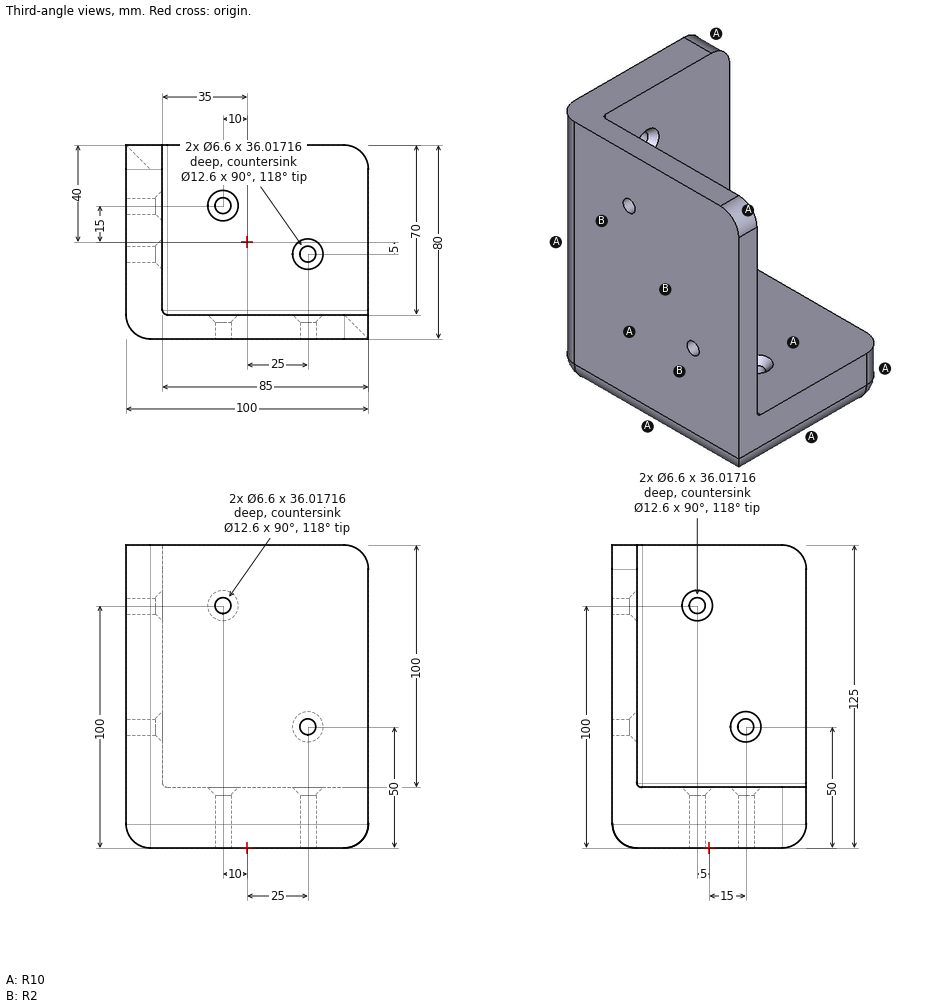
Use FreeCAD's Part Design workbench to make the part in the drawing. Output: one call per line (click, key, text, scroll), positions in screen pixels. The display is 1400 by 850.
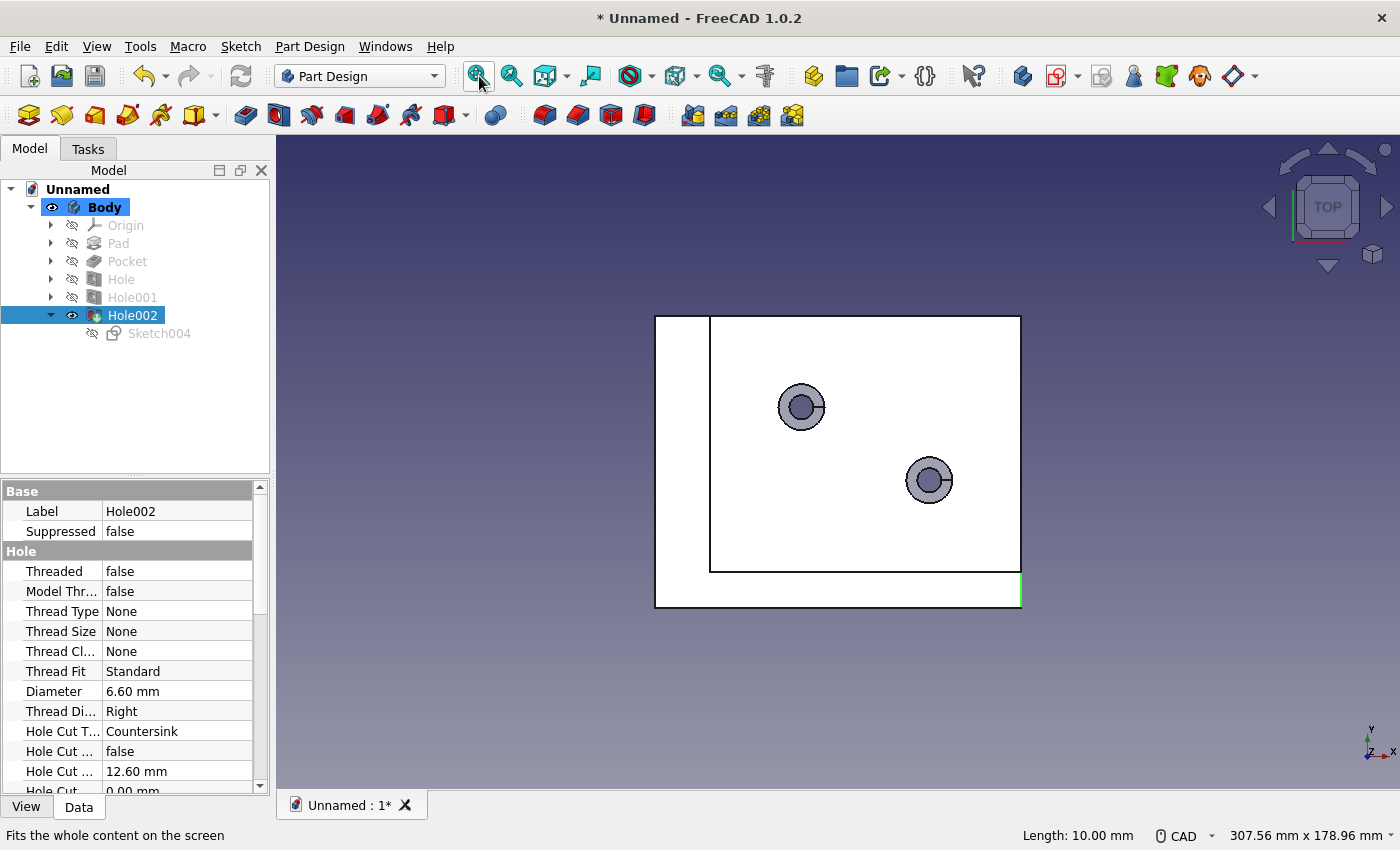
click(683, 315, ctrl)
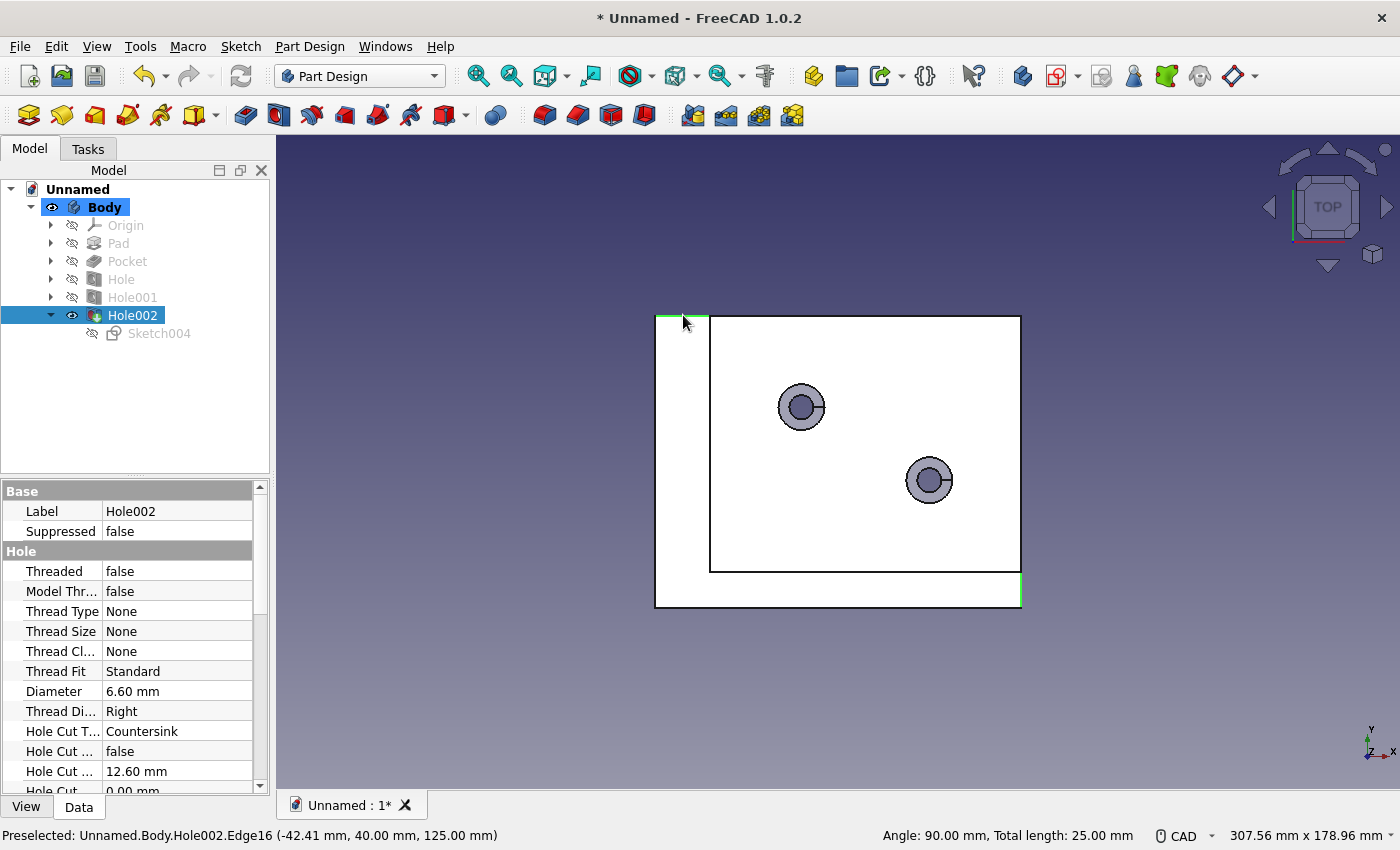
key(0)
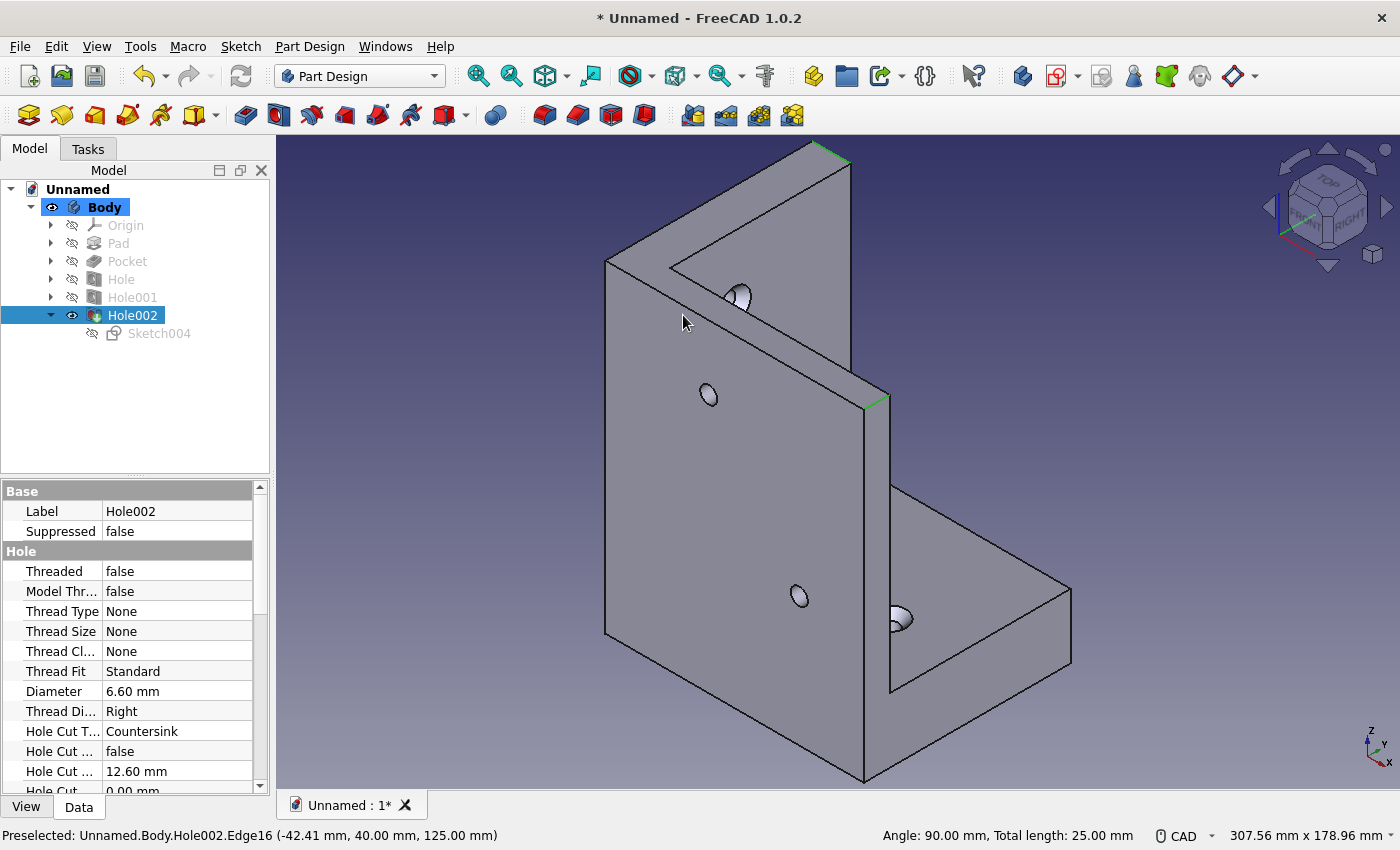
key(1)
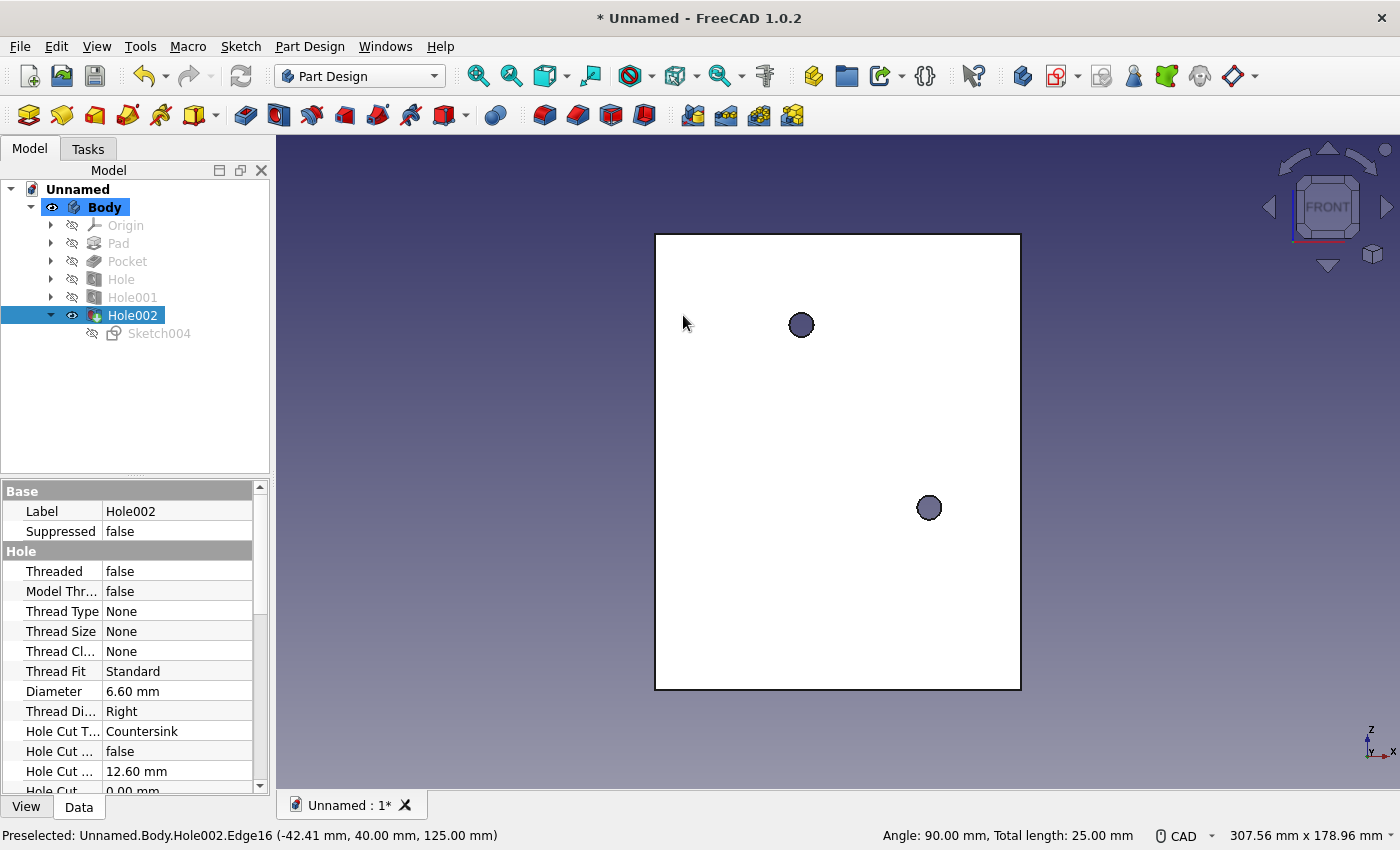
click(838, 689, ctrl)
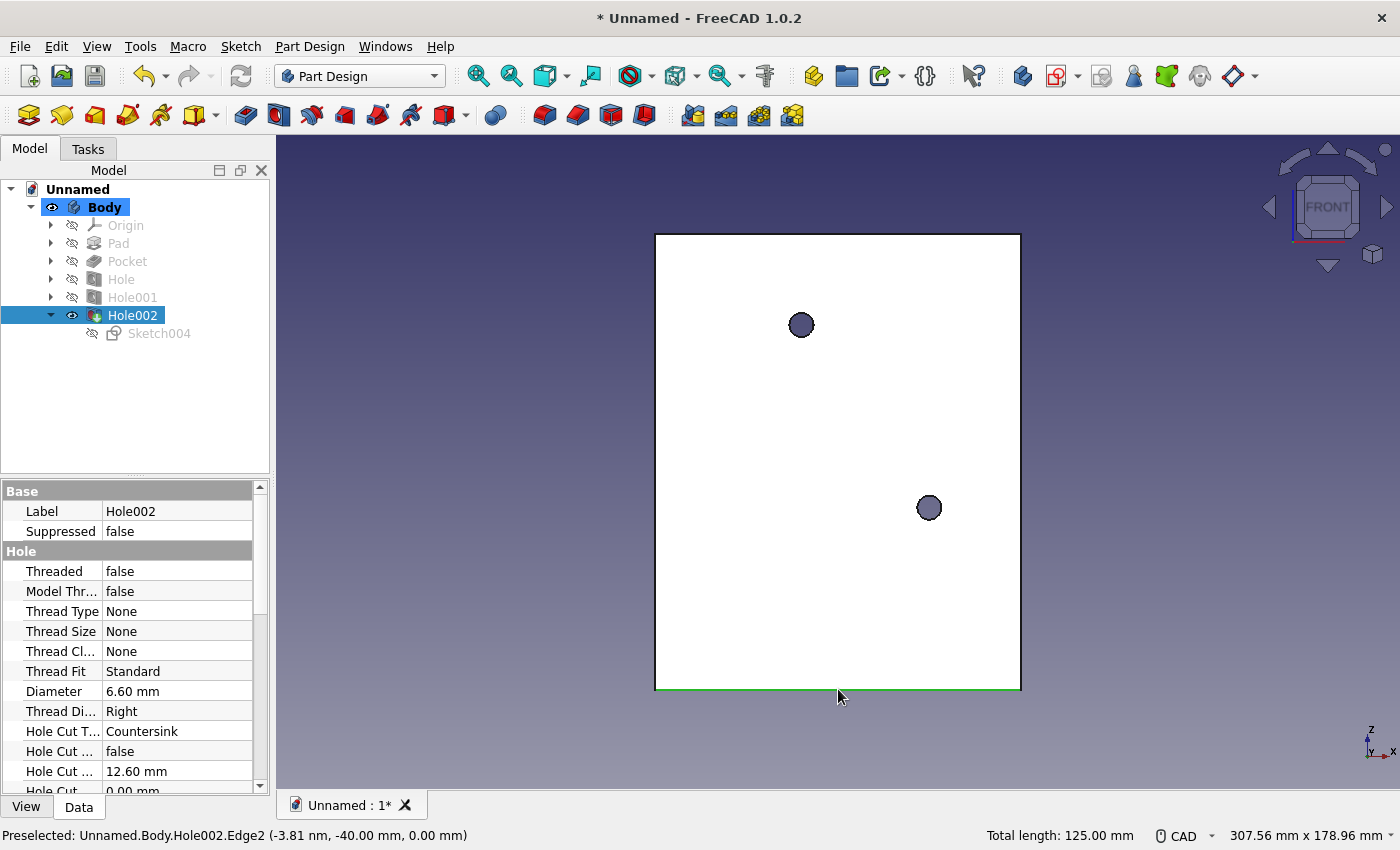
click(655, 461, ctrl)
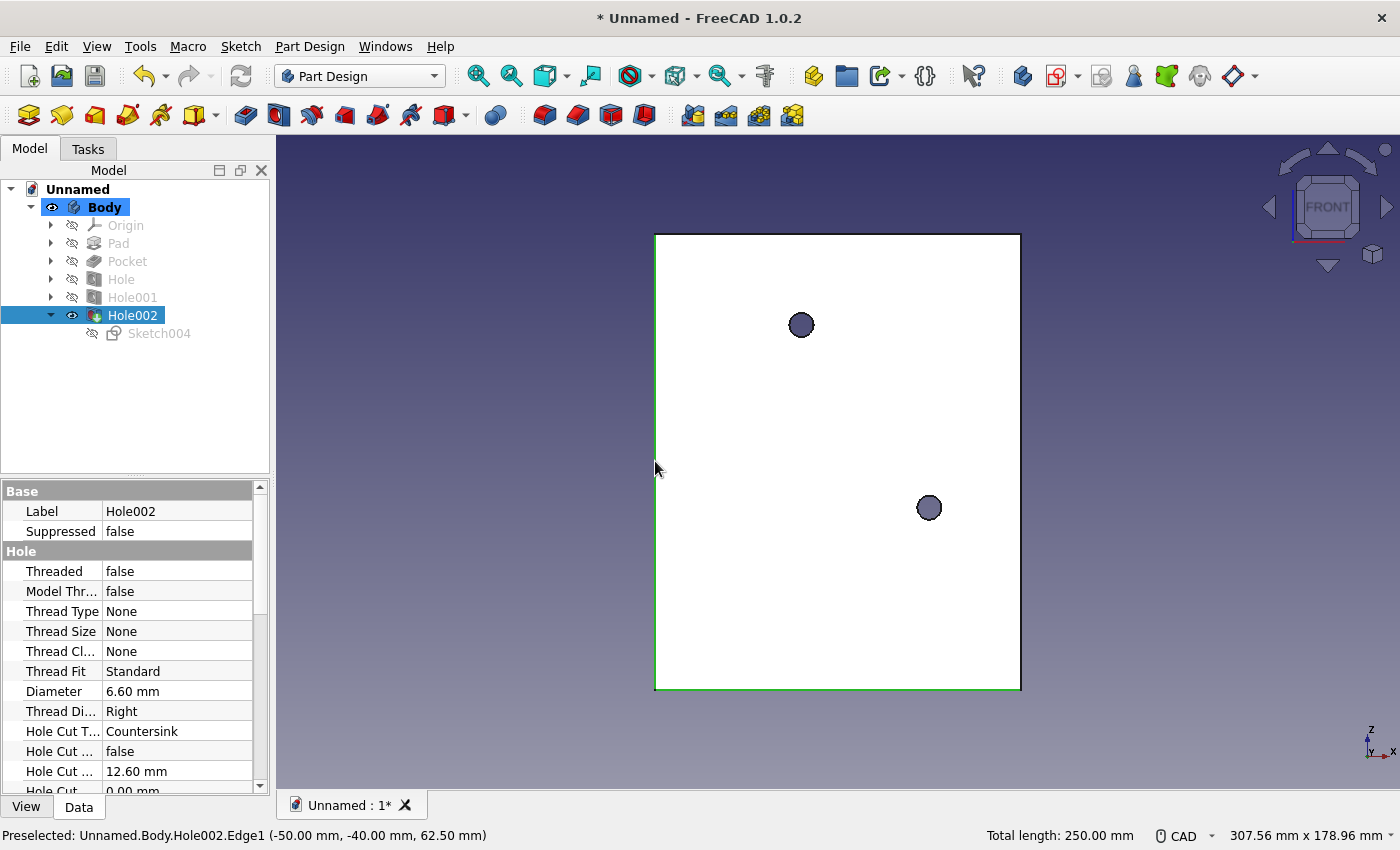
key(3)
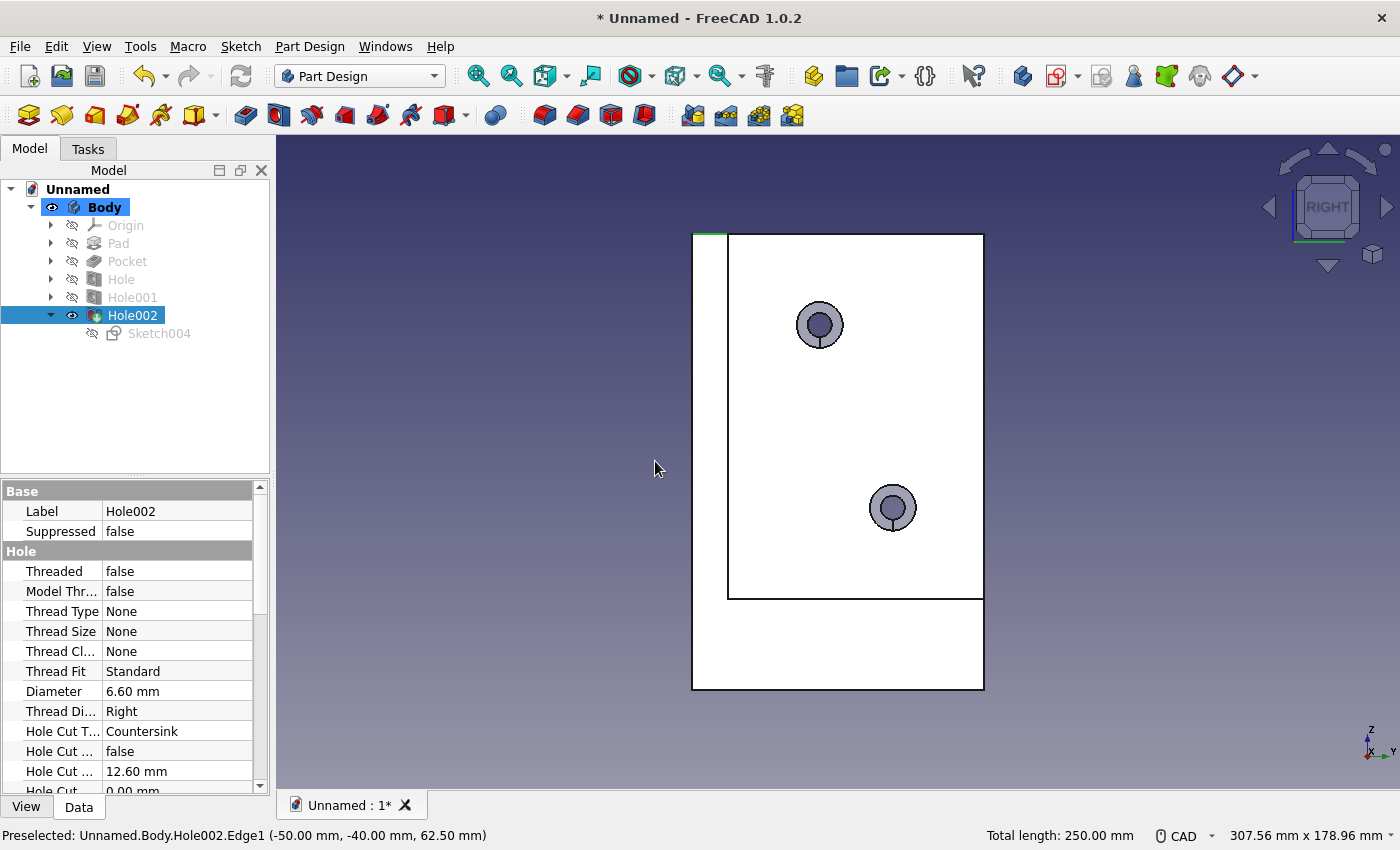
click(984, 644, ctrl)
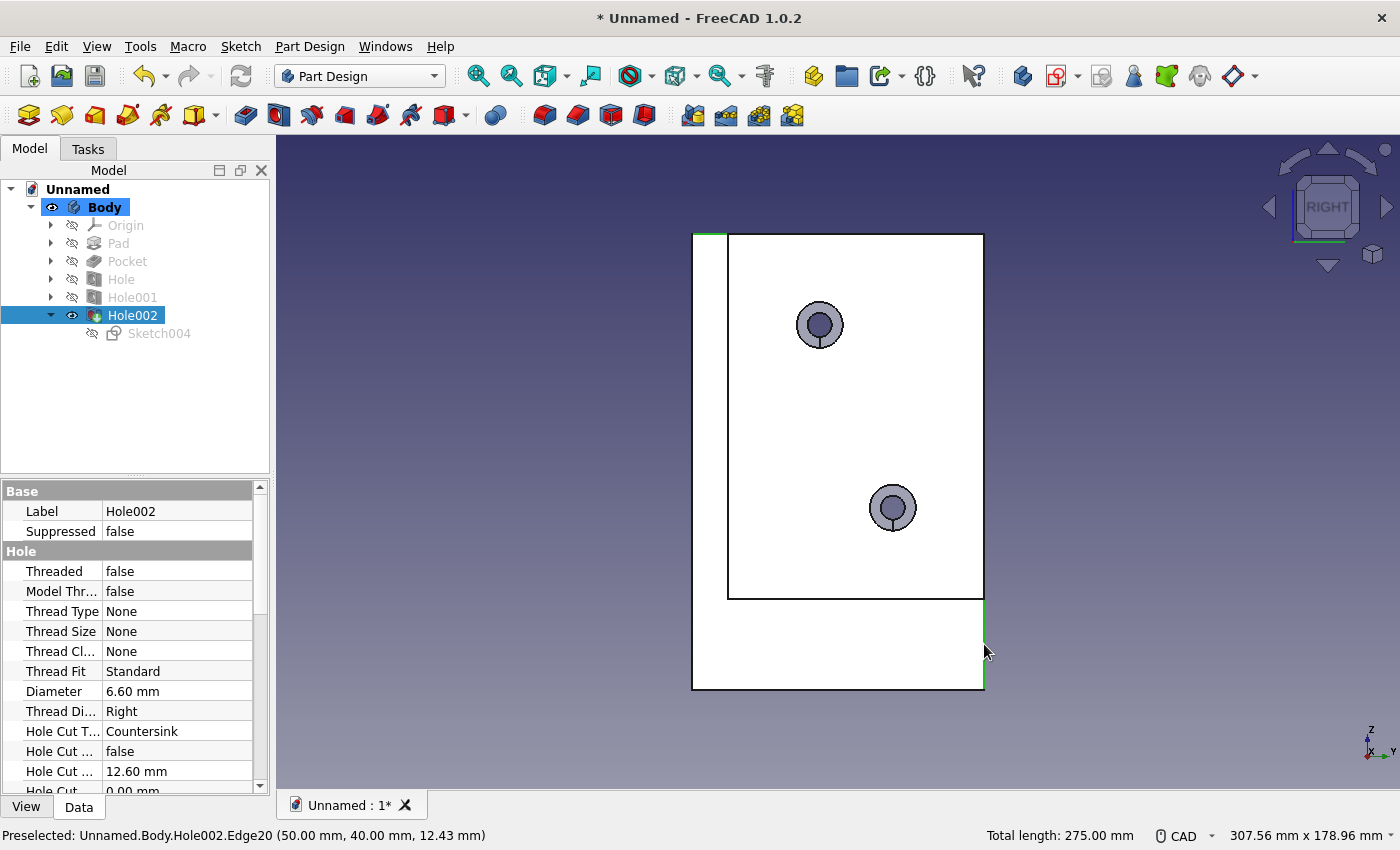
click(838, 689, ctrl)